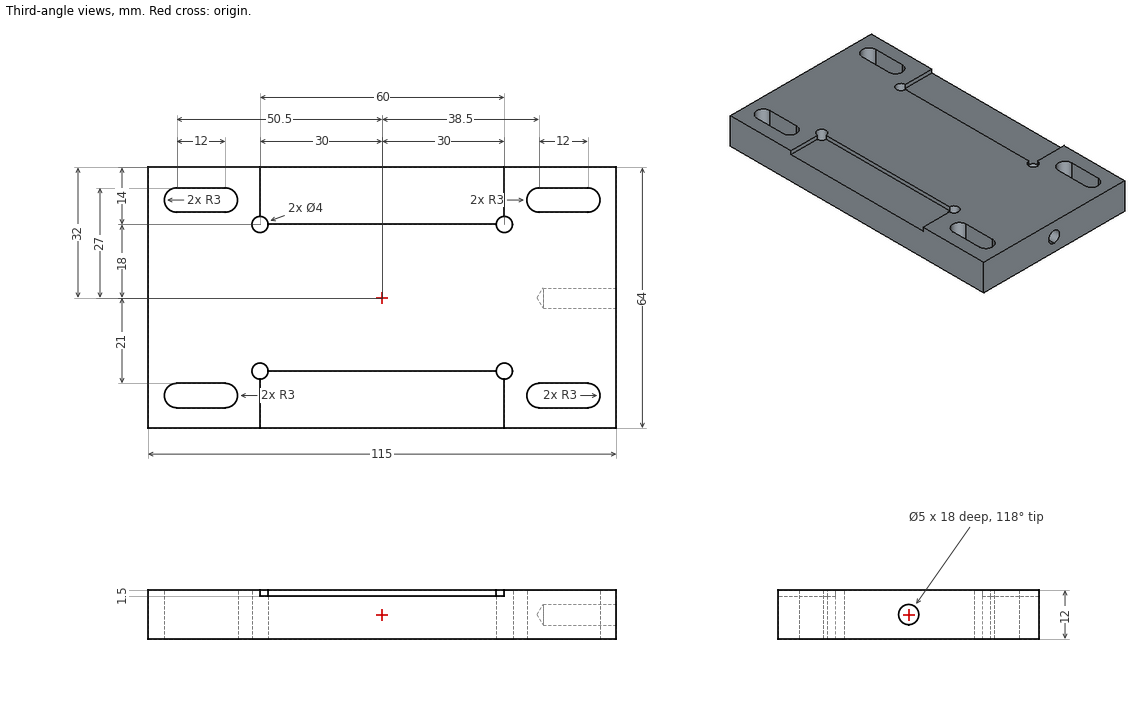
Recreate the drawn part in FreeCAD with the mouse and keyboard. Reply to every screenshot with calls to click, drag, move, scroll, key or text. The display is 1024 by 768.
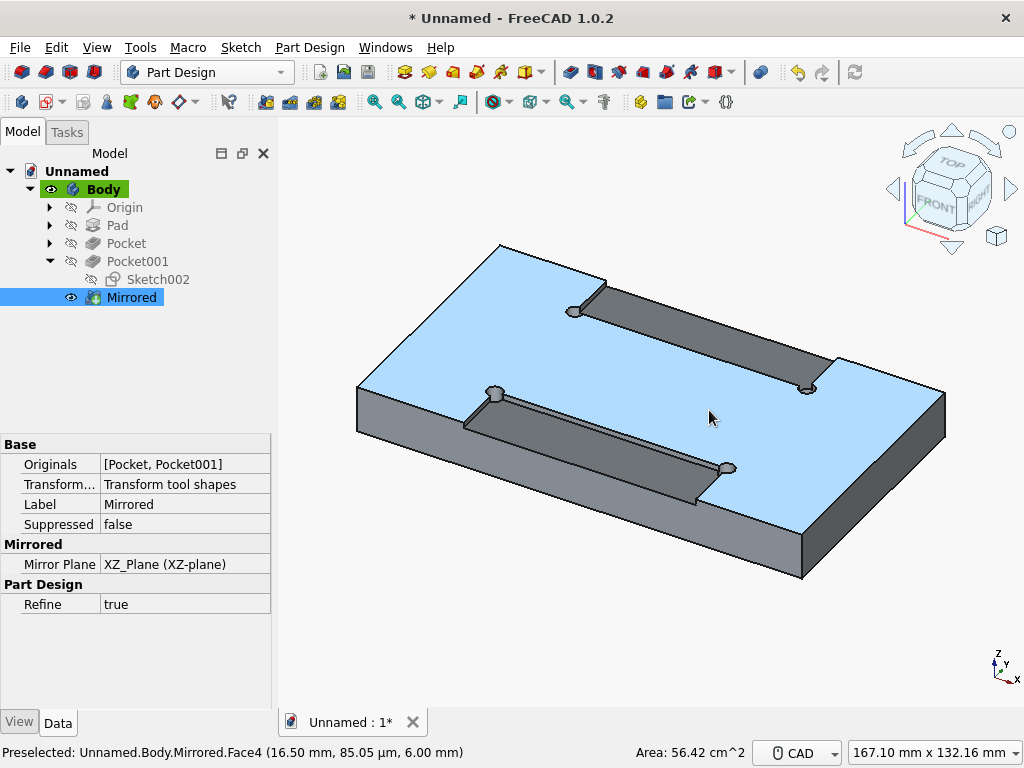
click(46, 102)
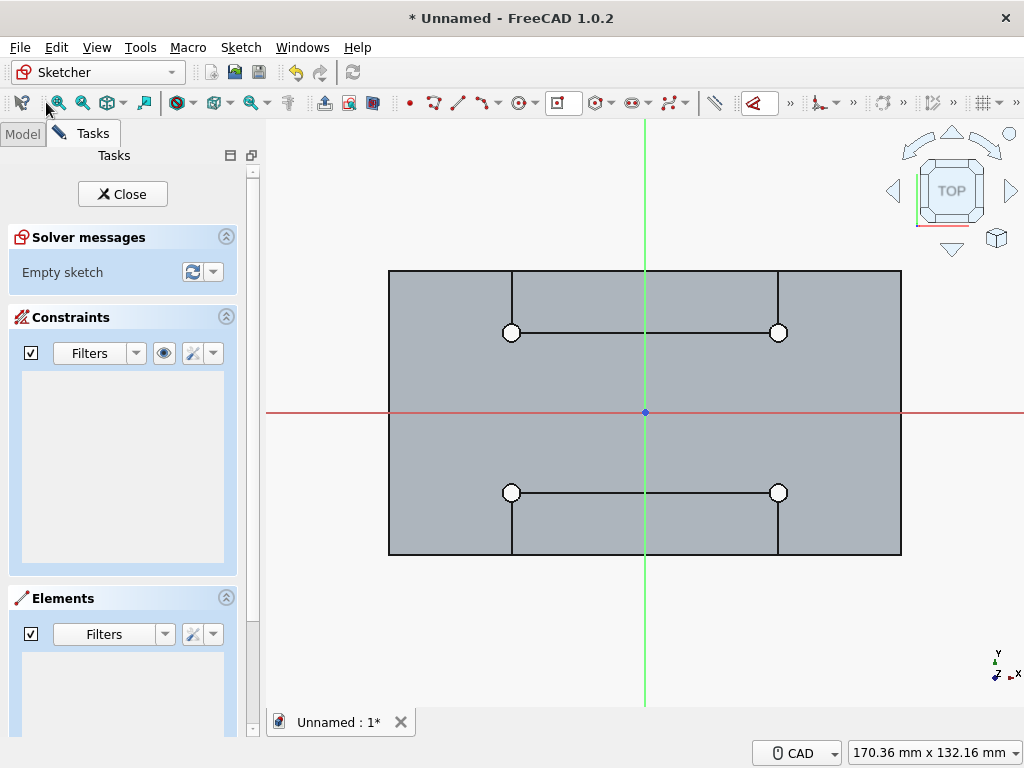
scroll(414, 279, up, 8)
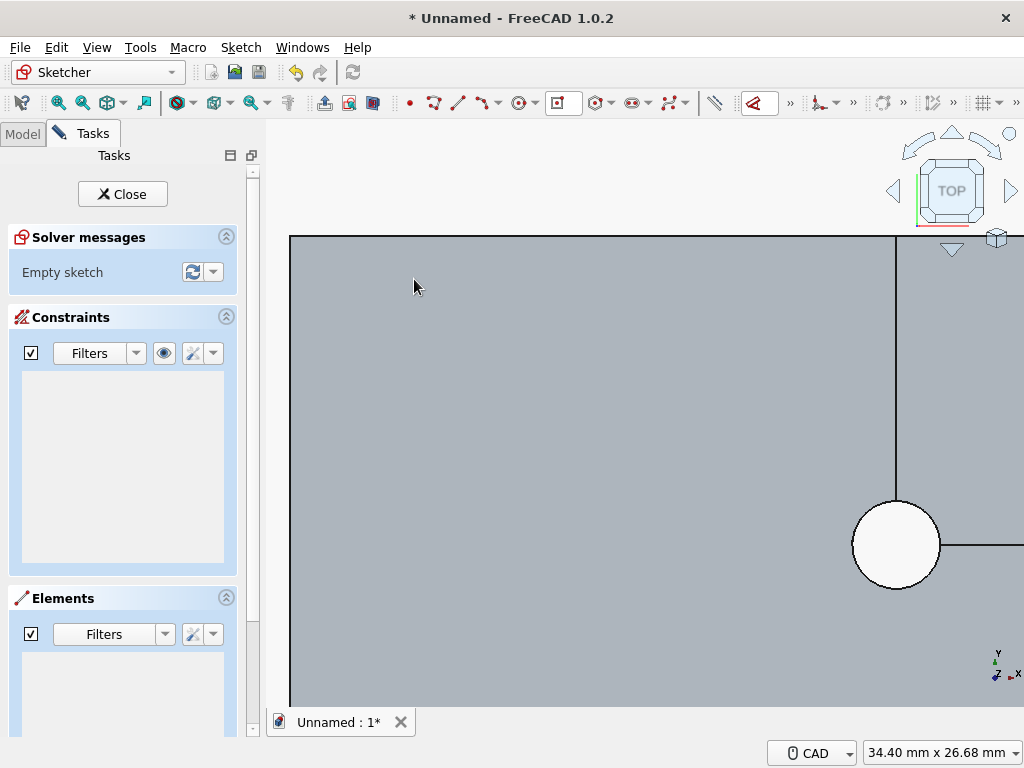
click(632, 104)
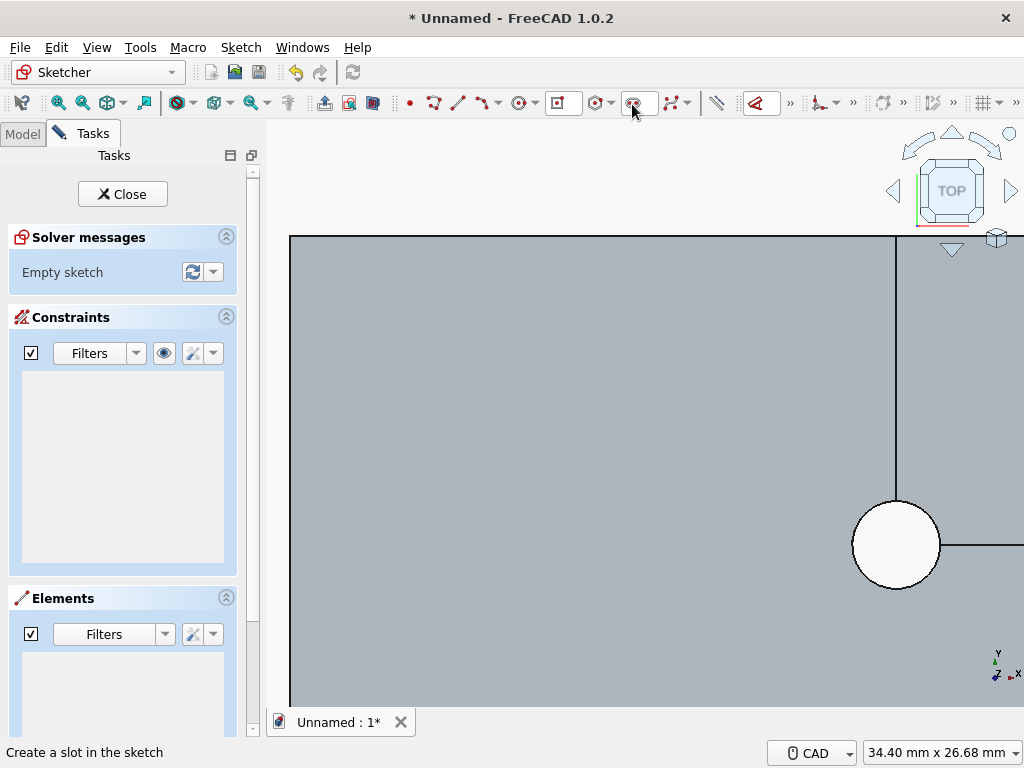
click(444, 413)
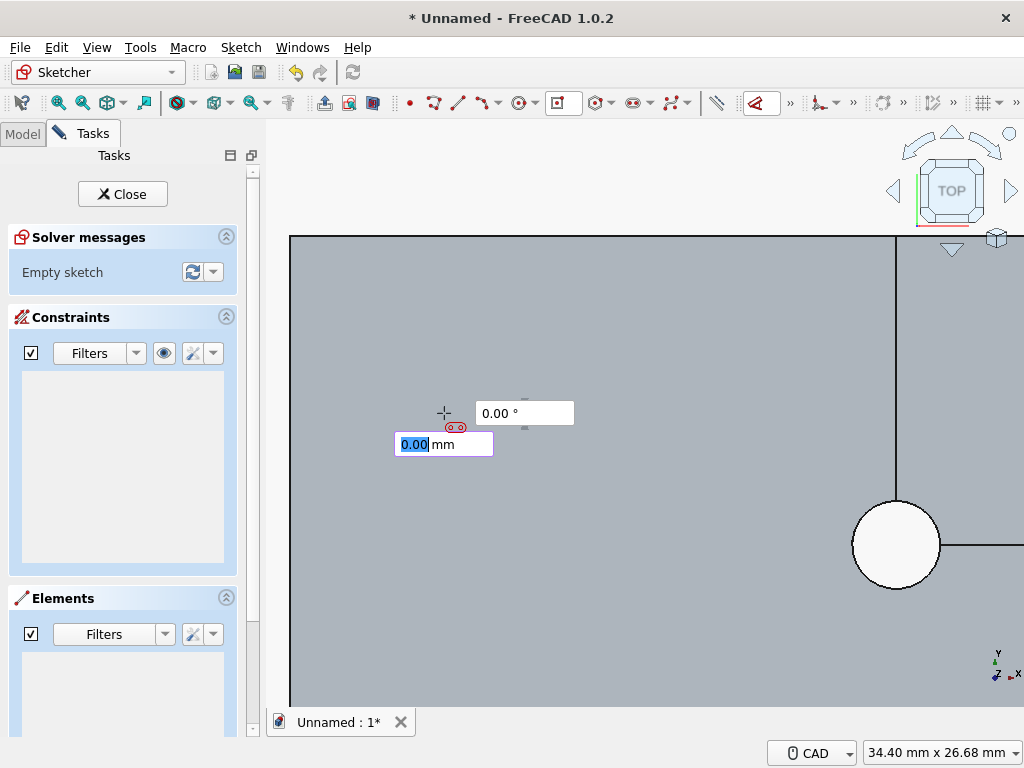
click(709, 413)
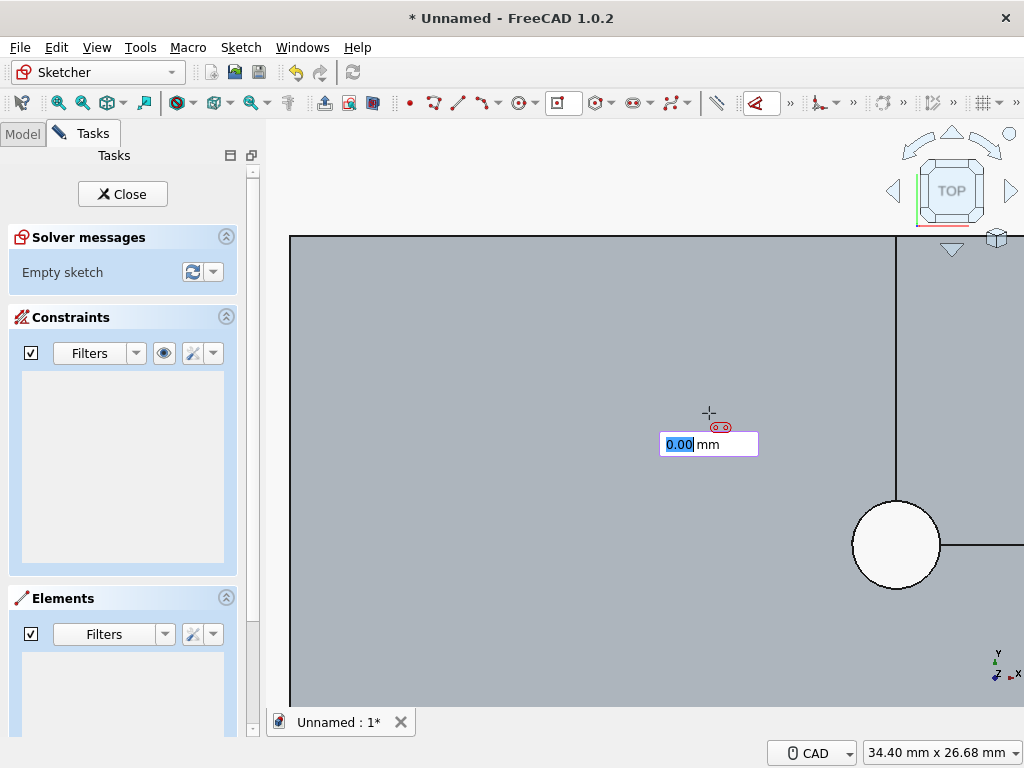
click(577, 347)
key(Escape)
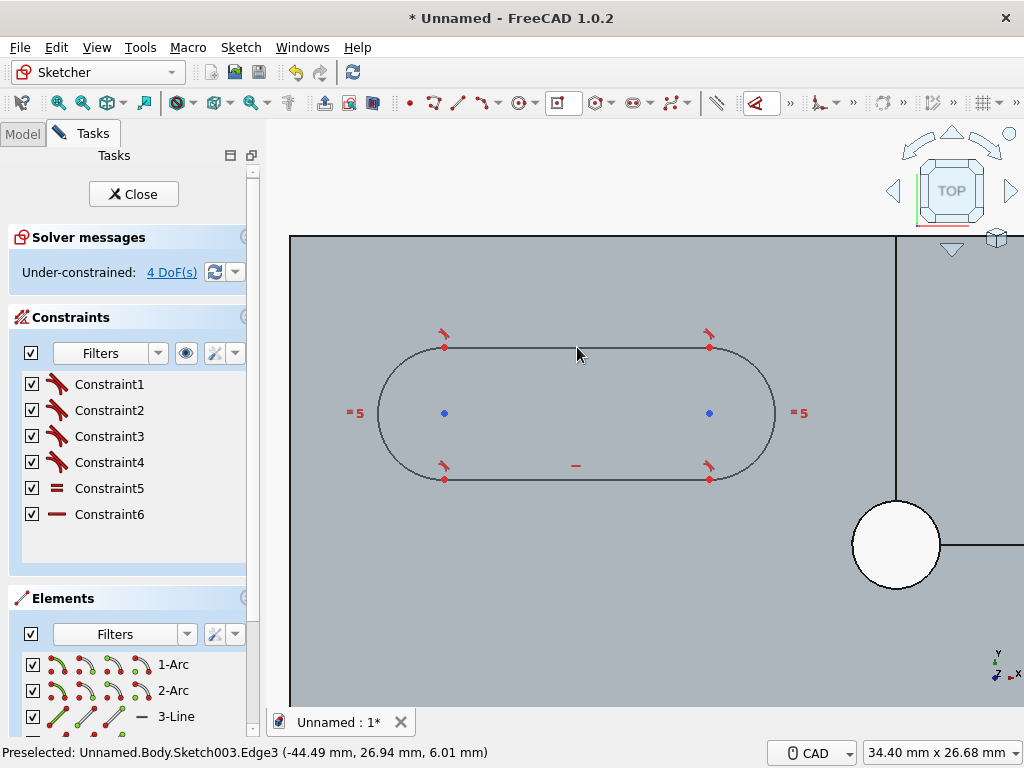
click(391, 375)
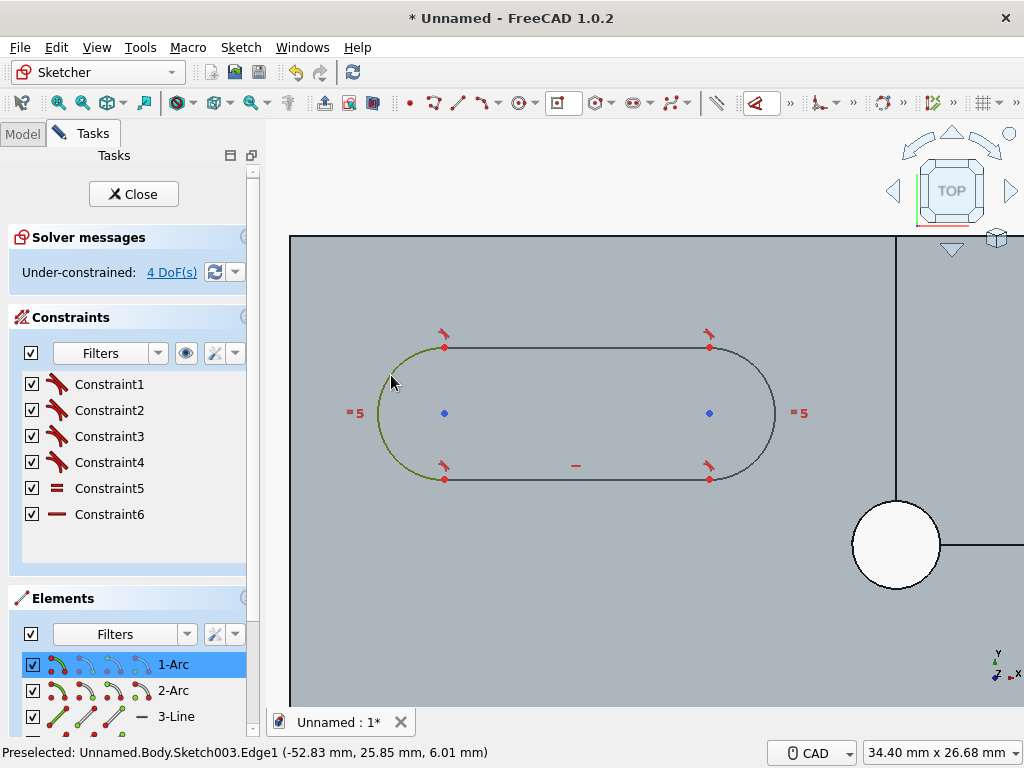
key(k)
key(r)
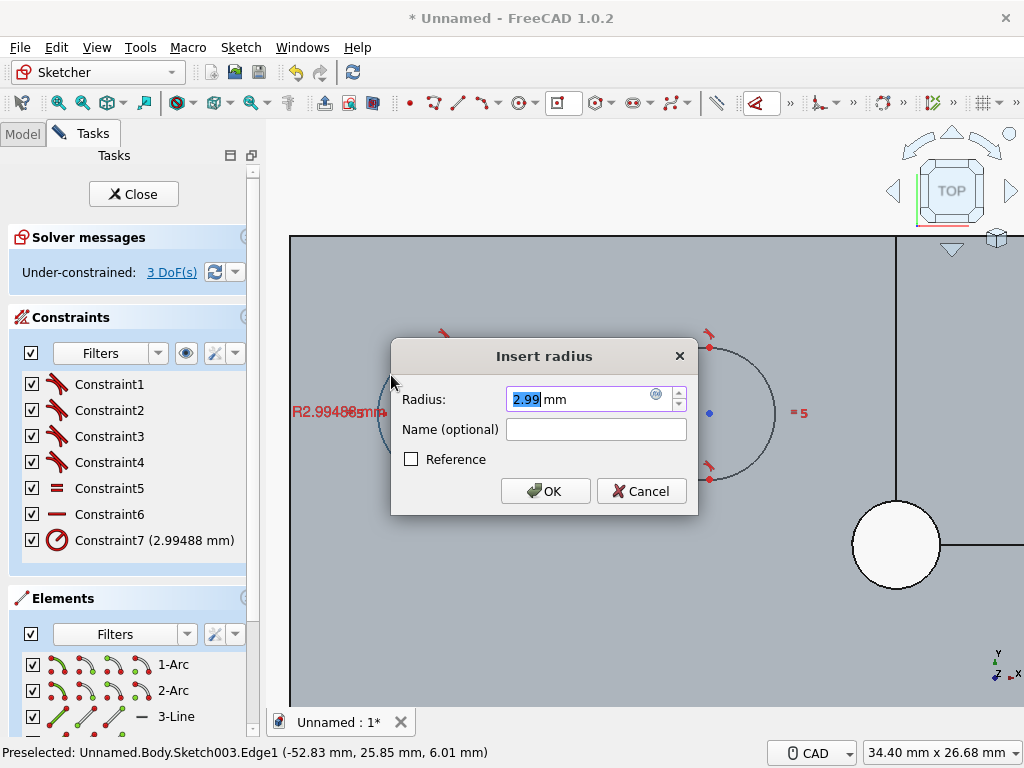
text(3)
key(Return)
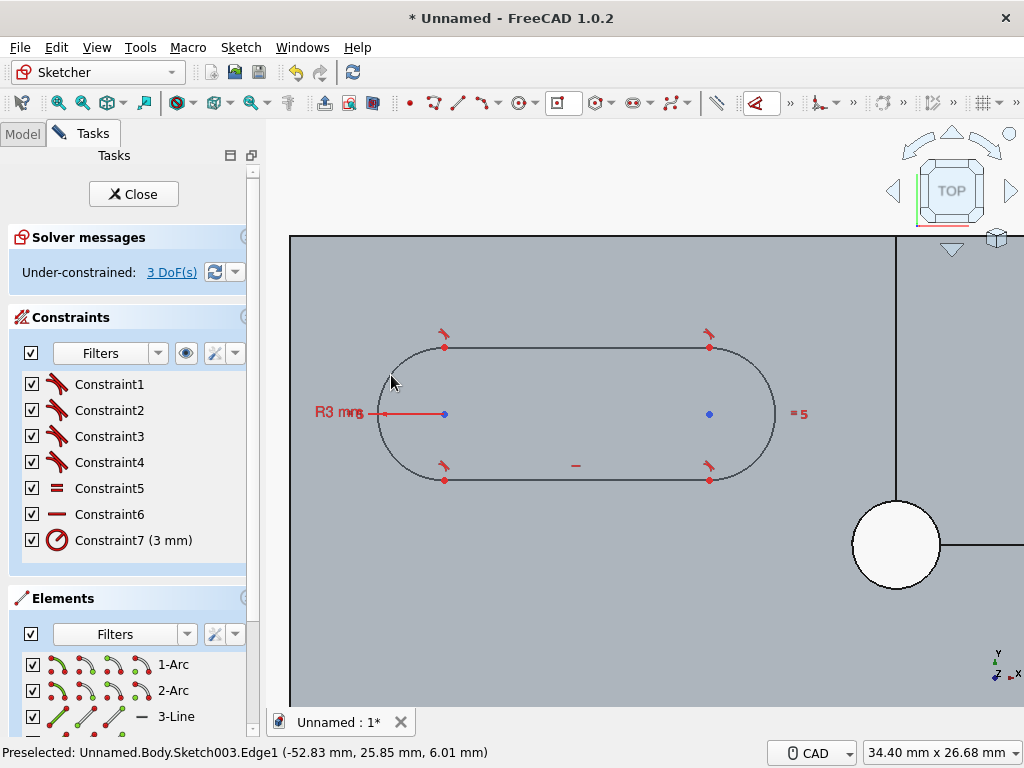
click(524, 348)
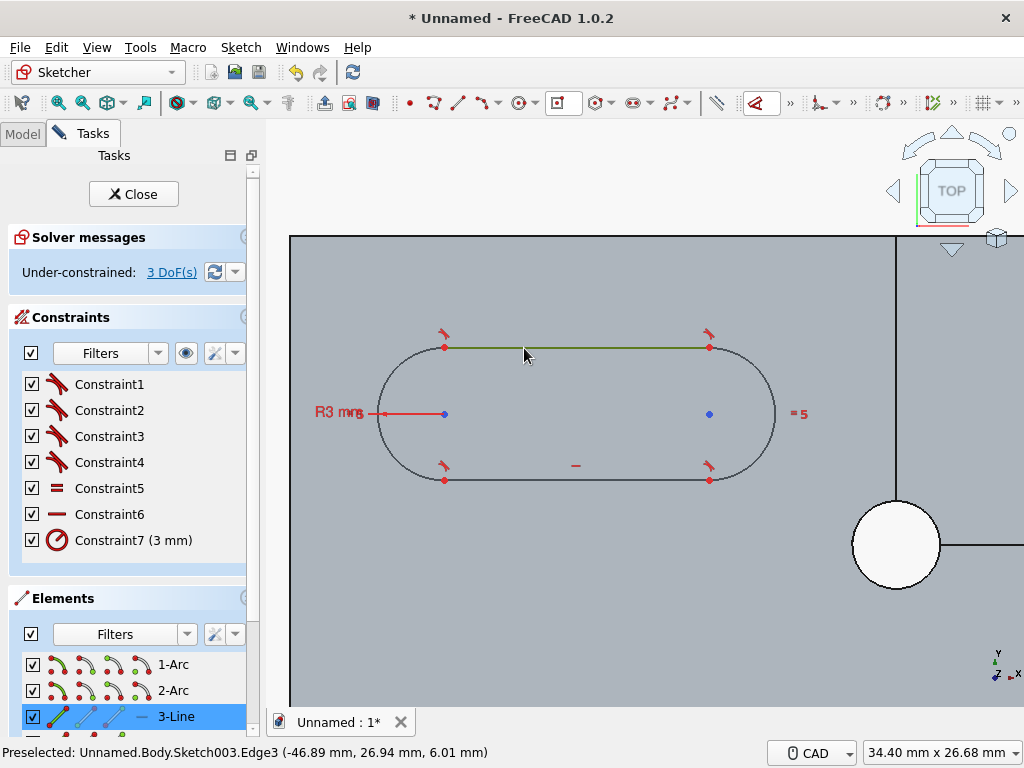
click(774, 104)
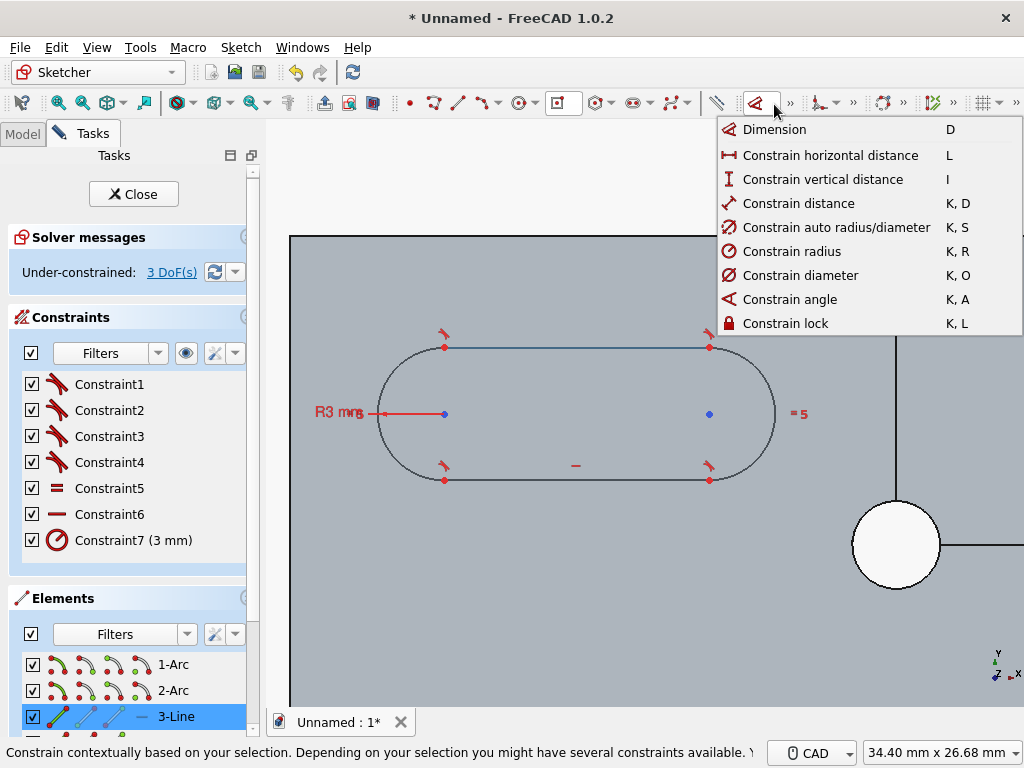
click(870, 155)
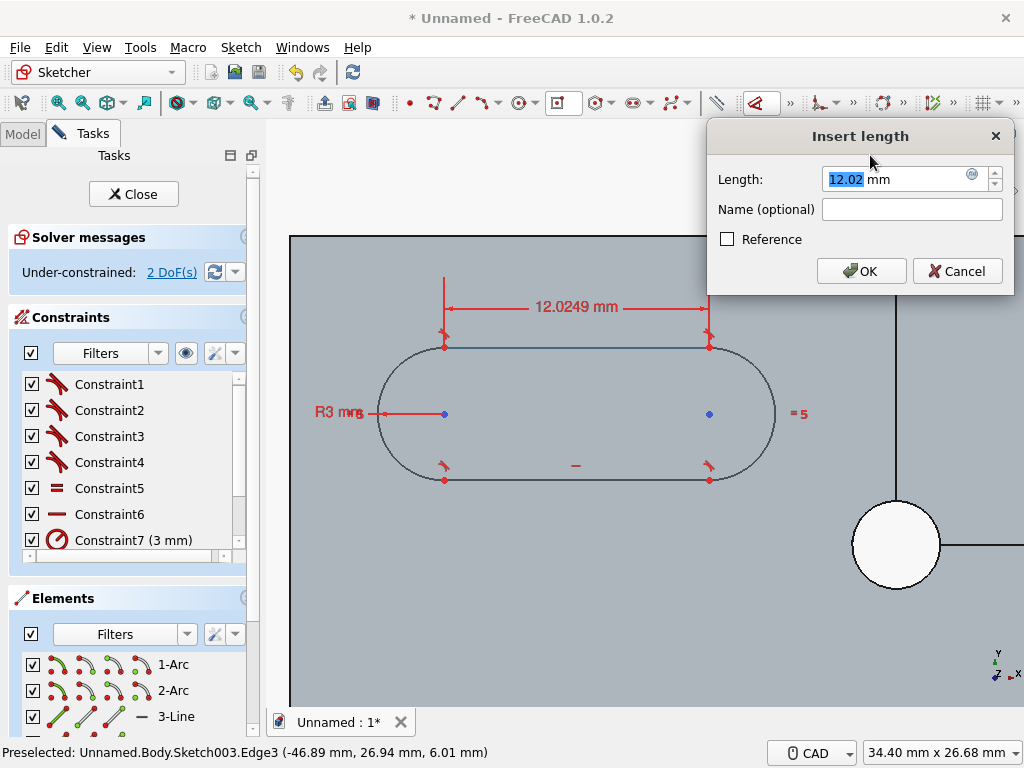
text(12)
key(Return)